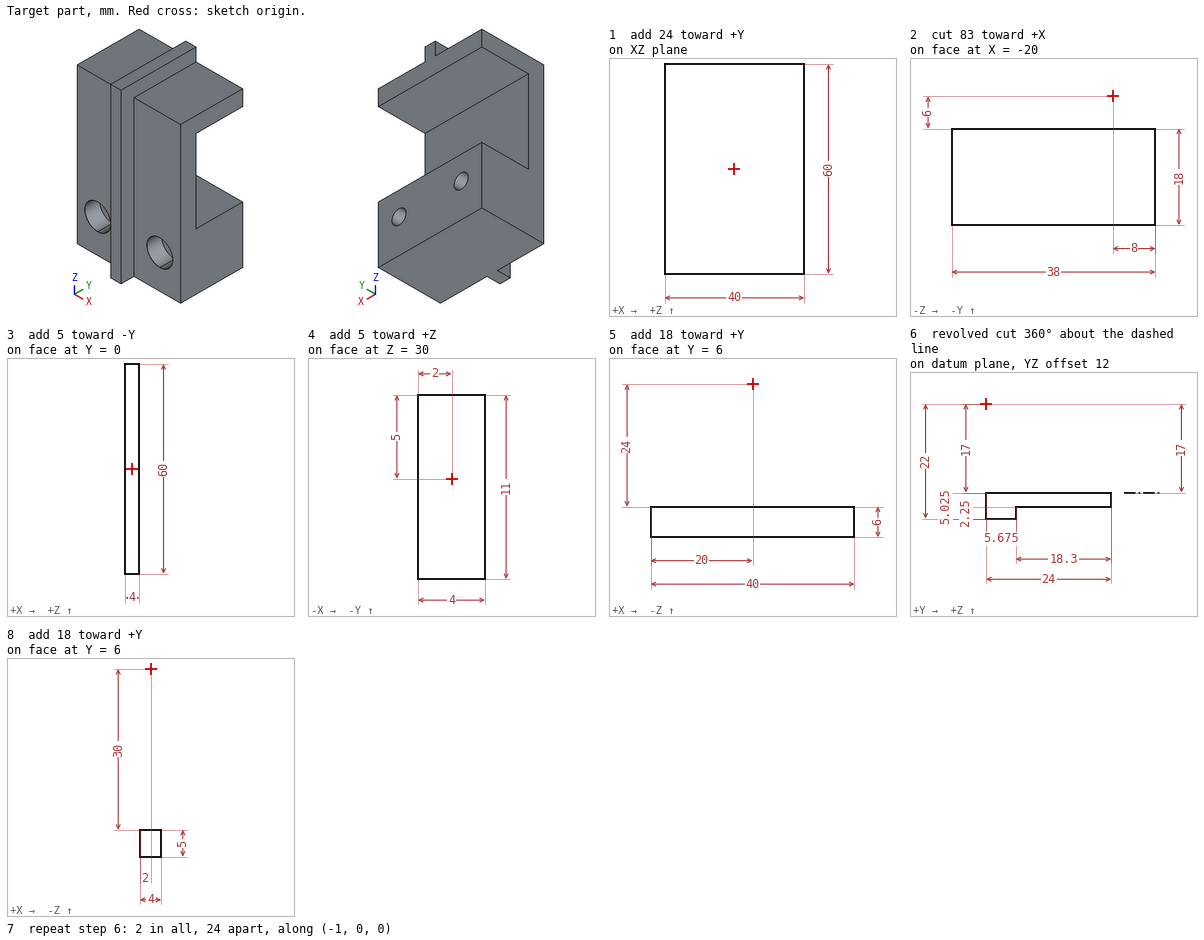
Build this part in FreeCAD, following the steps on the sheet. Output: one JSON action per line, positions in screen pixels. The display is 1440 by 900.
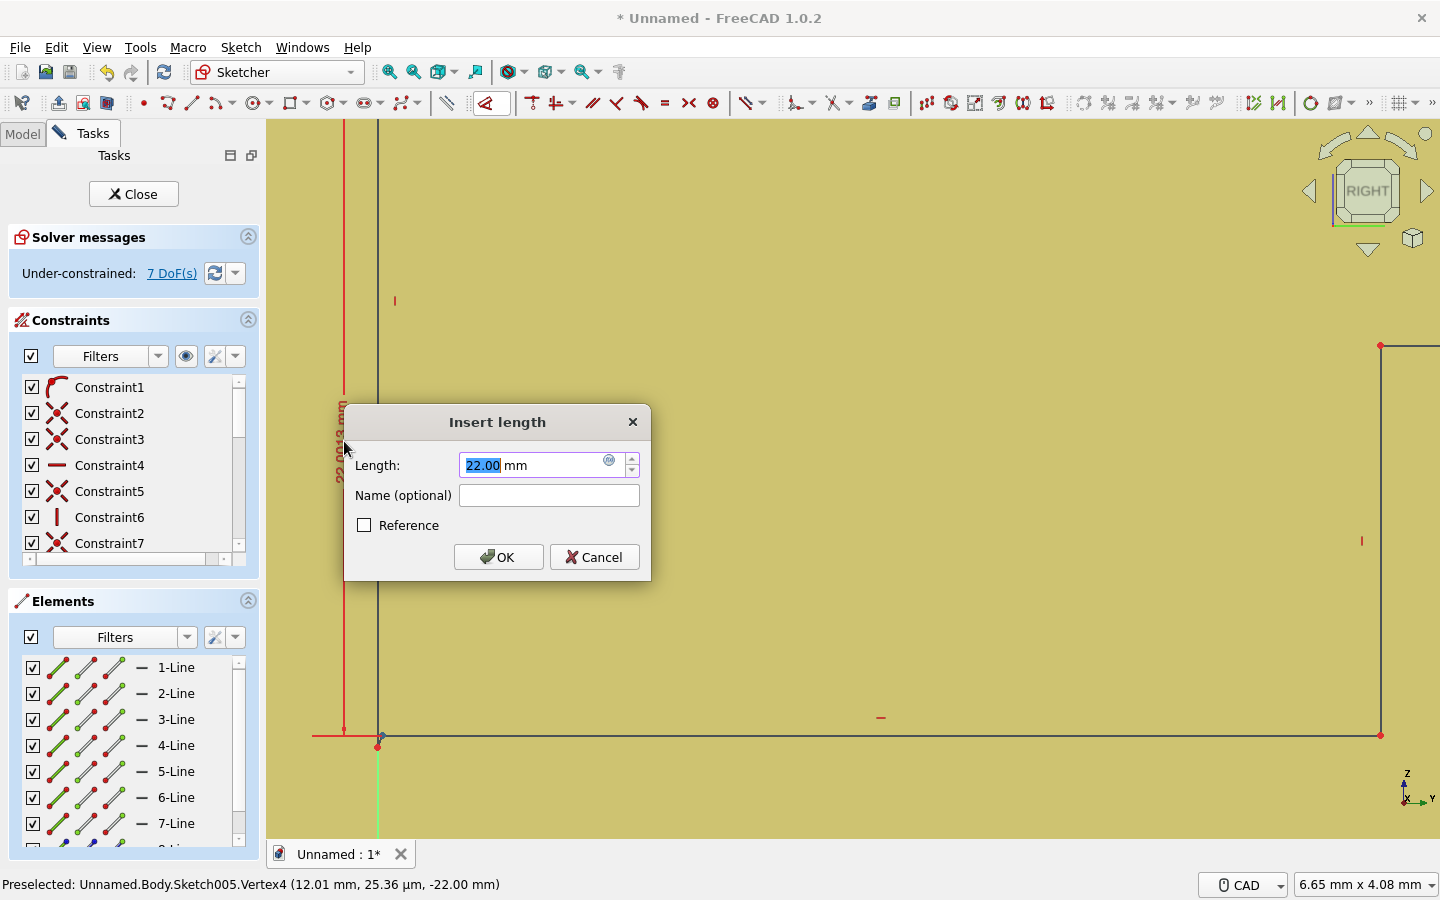
{"action": "type", "text": "22"}
{"action": "key", "text": "Return"}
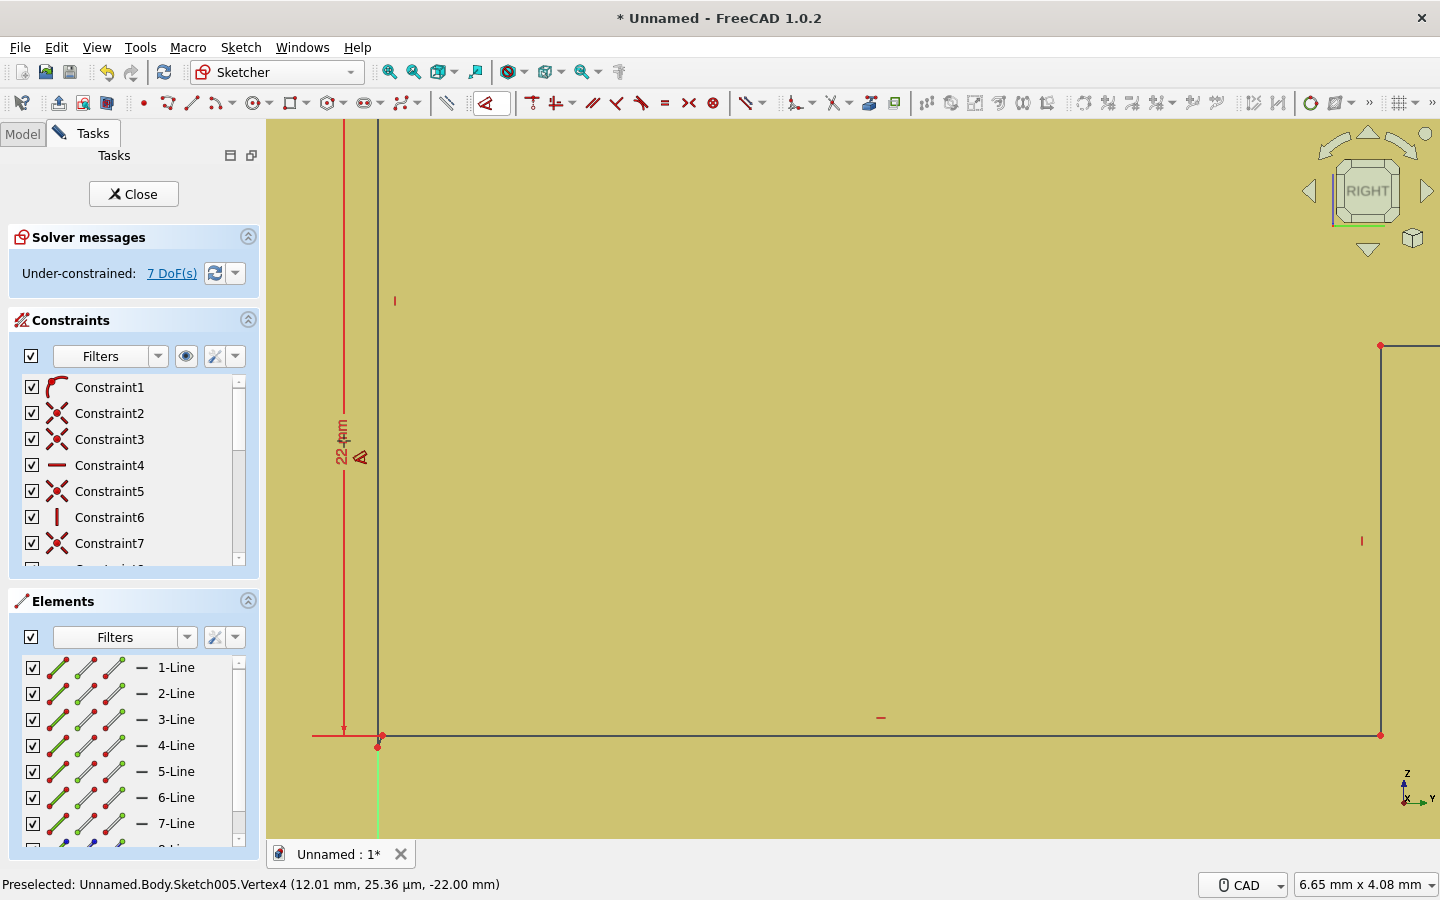
{"action": "scroll", "coordinate": [465, 689], "scroll_direction": "down", "scroll_amount": 11}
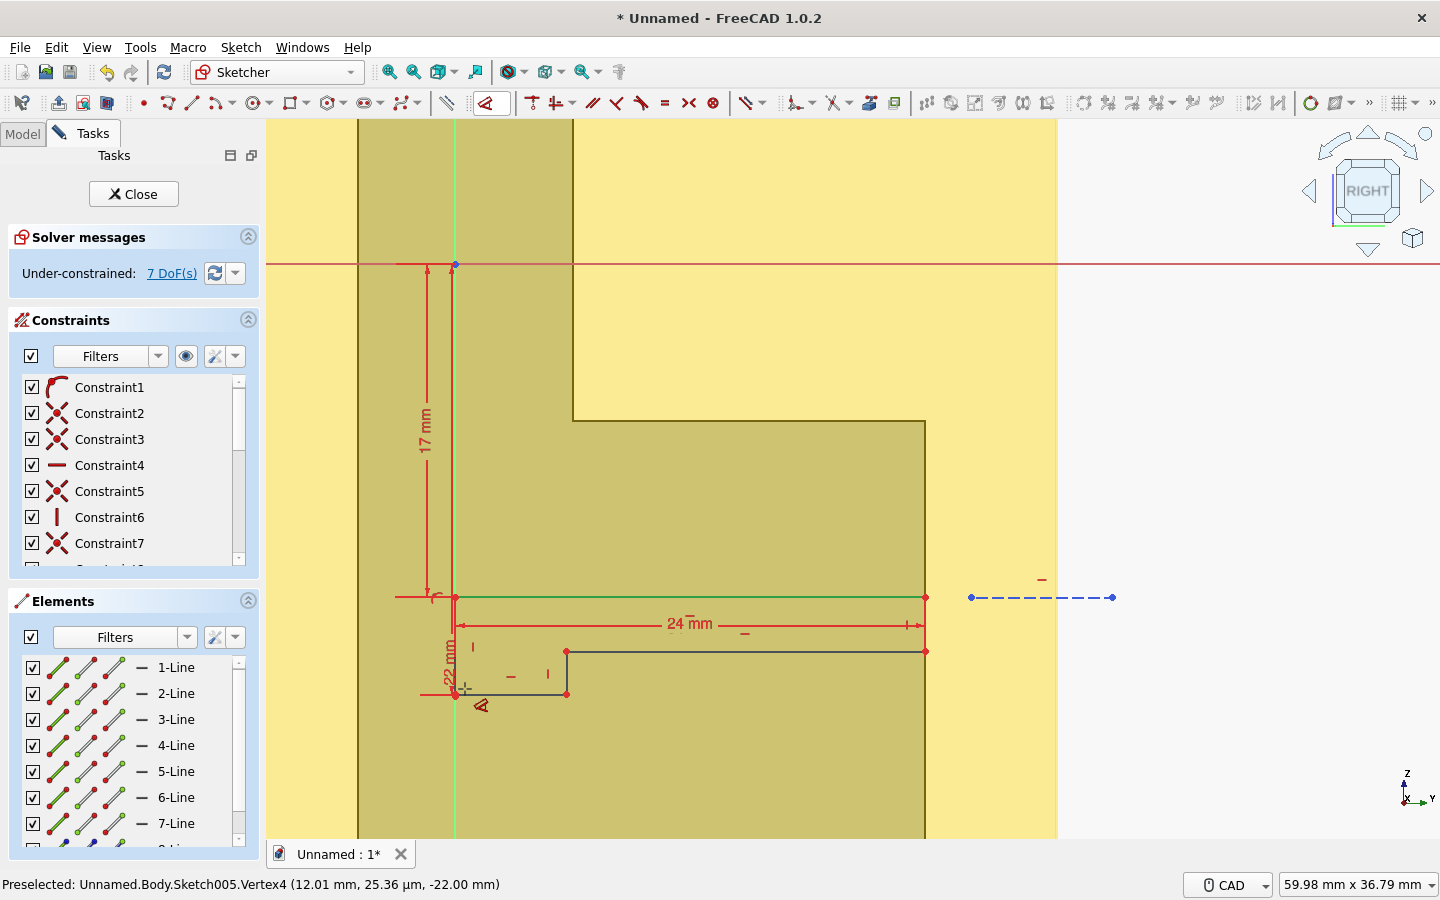
{"action": "left_click", "coordinate": [972, 598]}
{"action": "left_click", "coordinate": [421, 354]}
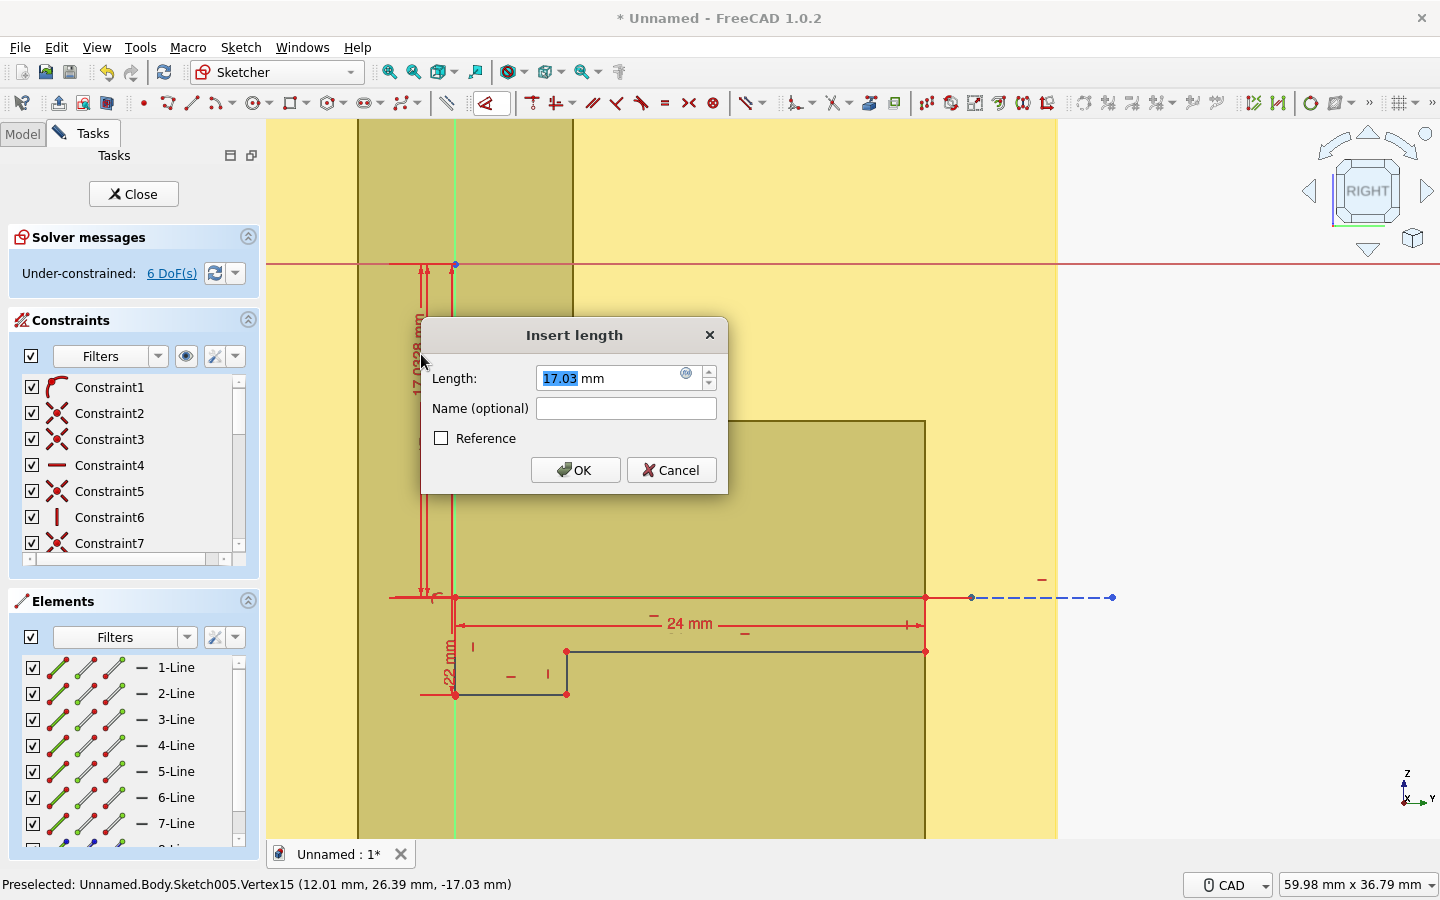
{"action": "type", "text": "17"}
{"action": "key", "text": "Return"}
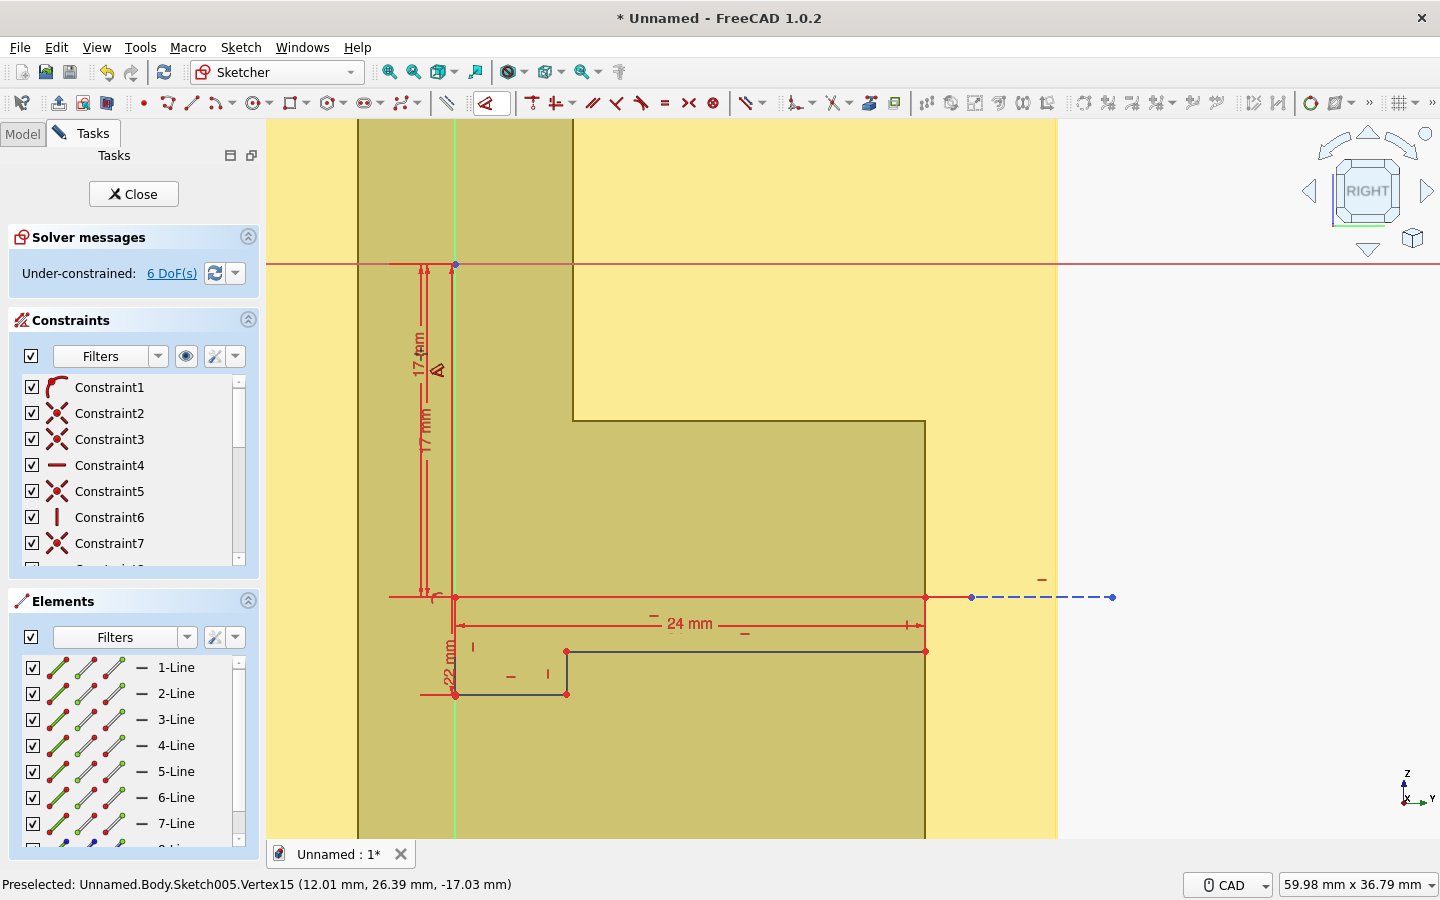
{"action": "left_click", "coordinate": [567, 682]}
{"action": "left_click", "coordinate": [533, 673]}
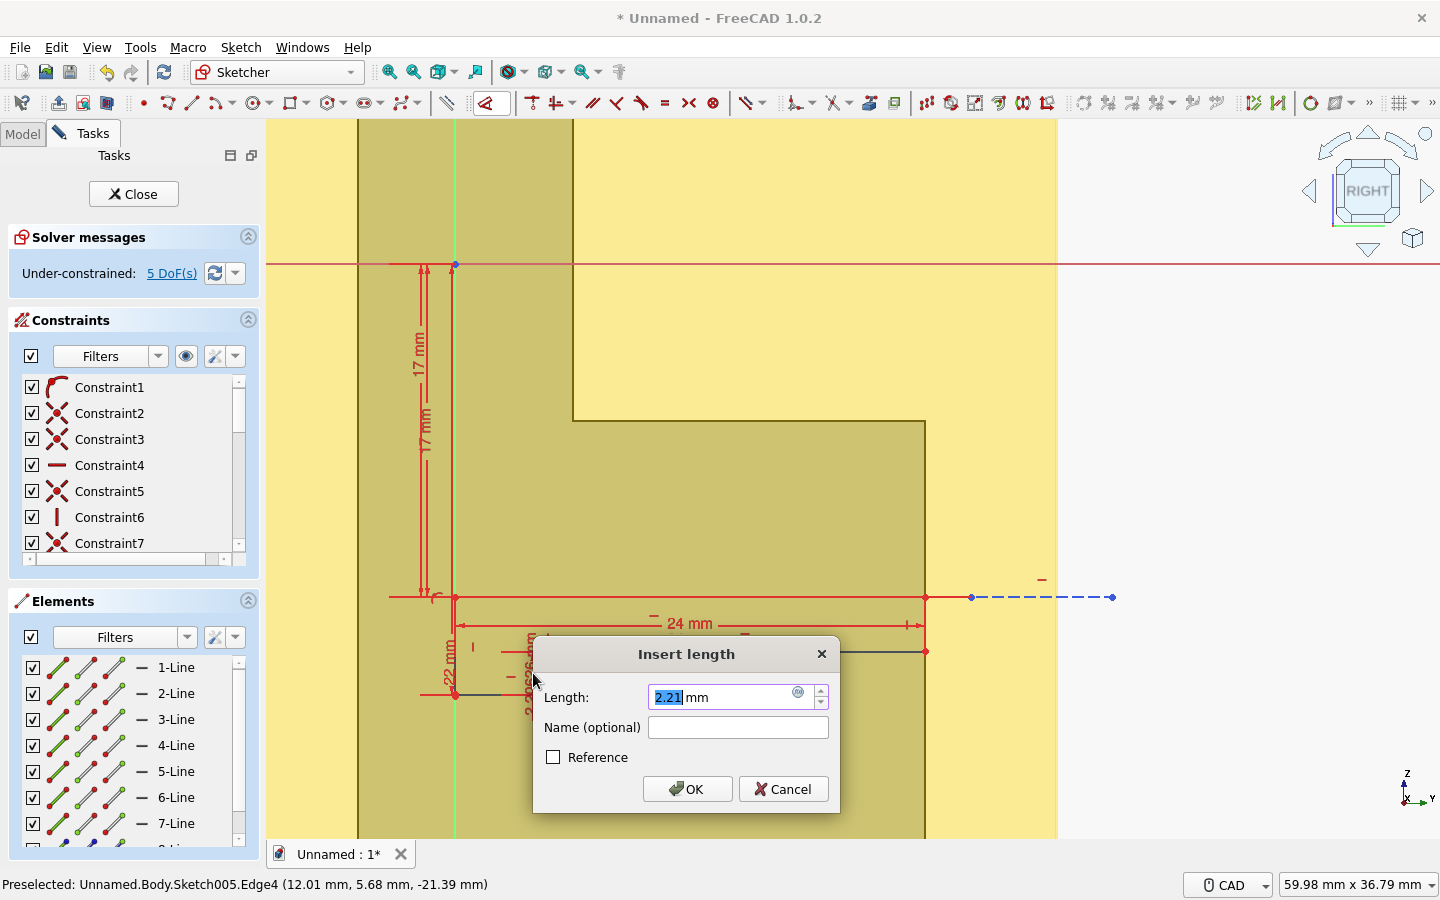
{"action": "type", "text": "2.25"}
{"action": "key", "text": "Return"}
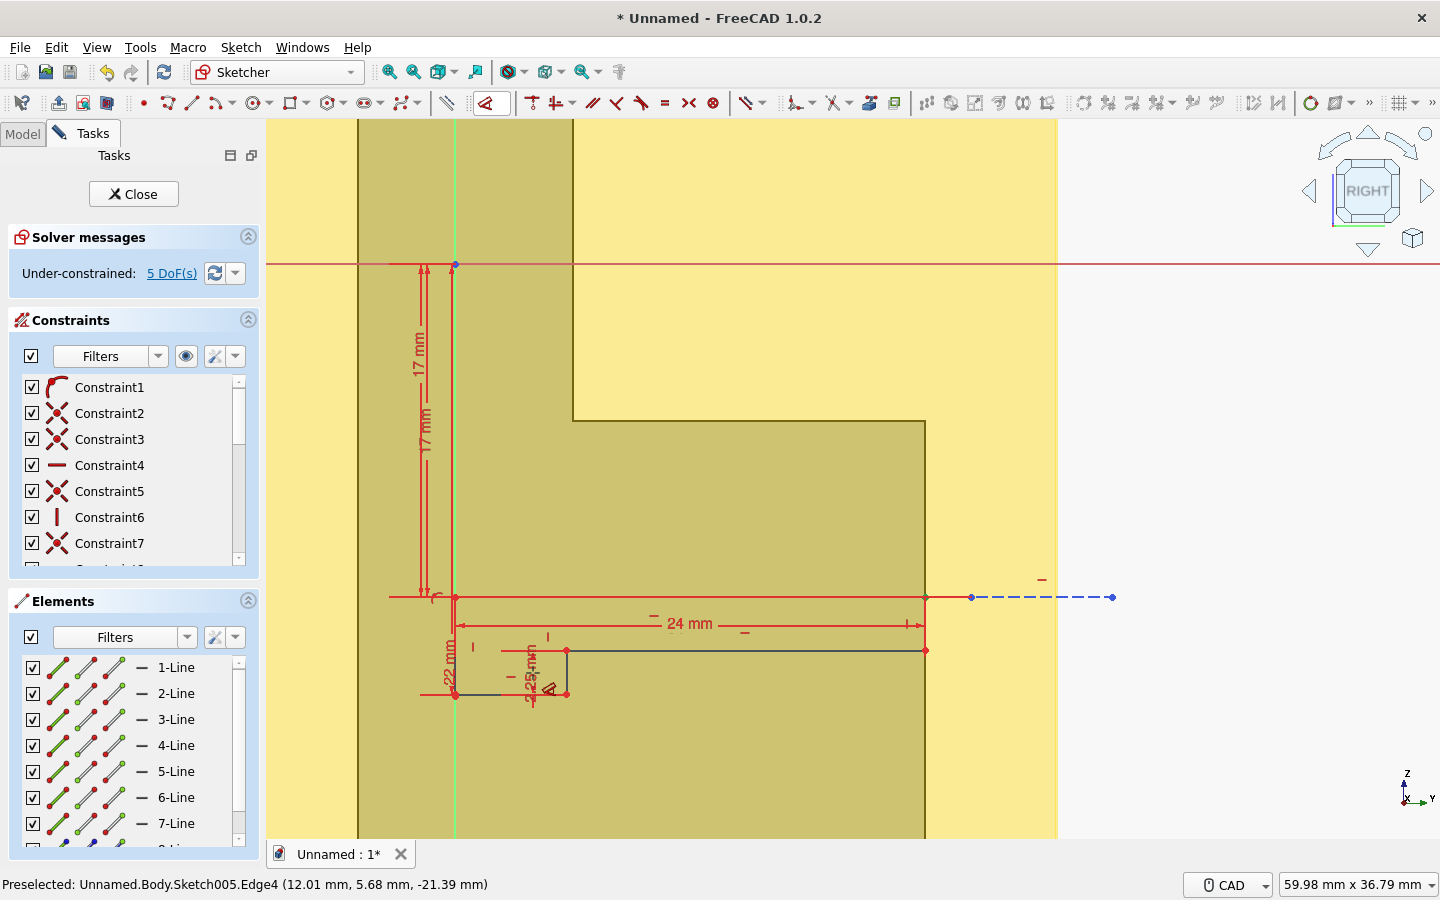
{"action": "left_click", "coordinate": [674, 651]}
{"action": "left_click", "coordinate": [746, 685]}